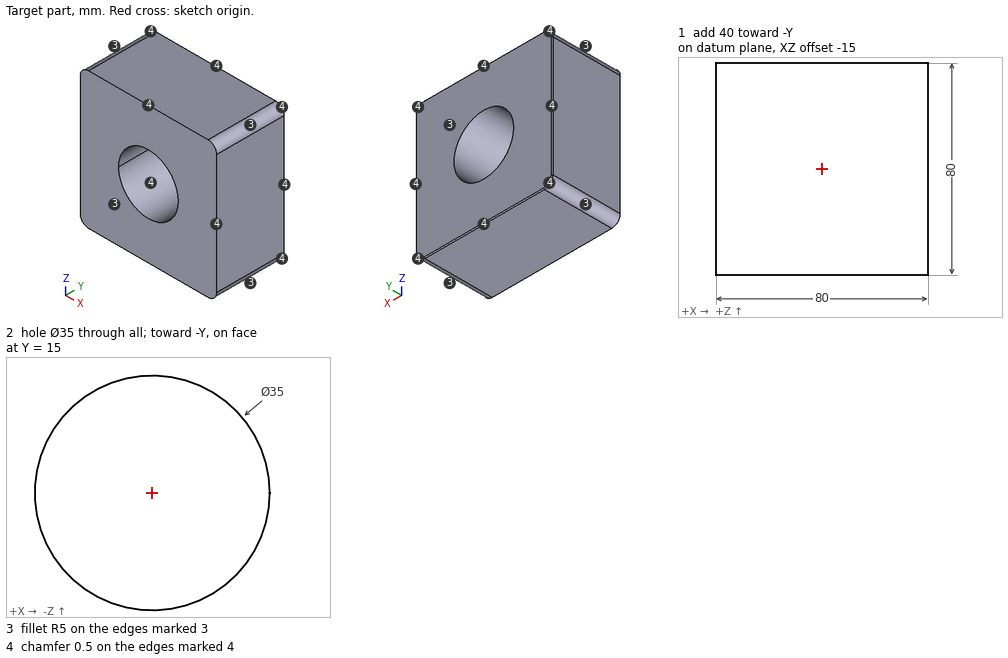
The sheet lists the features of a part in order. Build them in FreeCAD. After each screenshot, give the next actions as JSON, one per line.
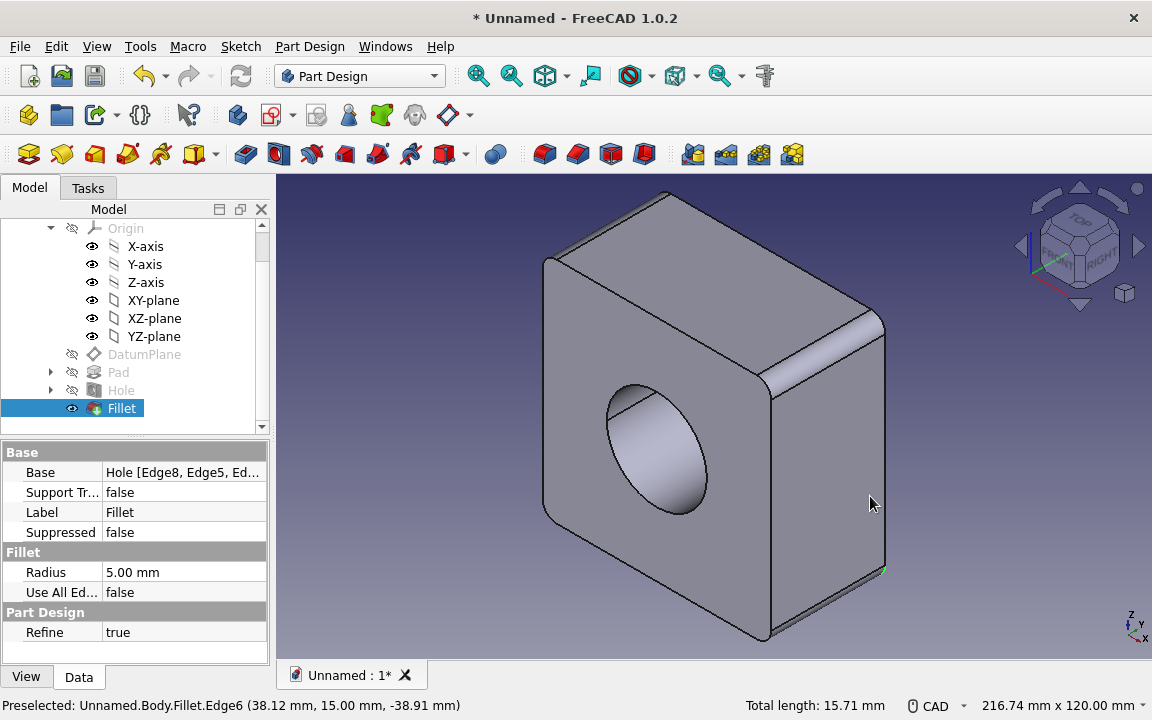
{"action": "left_click", "coordinate": [885, 327], "text": "ctrl"}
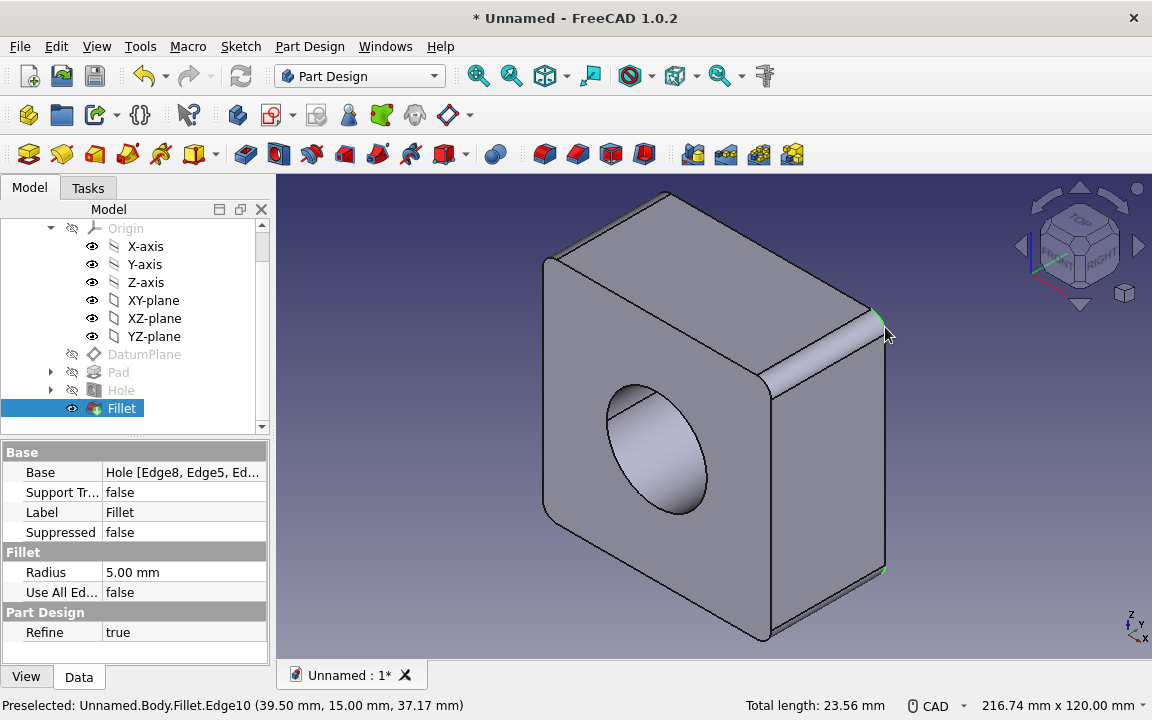
{"action": "key", "text": "2"}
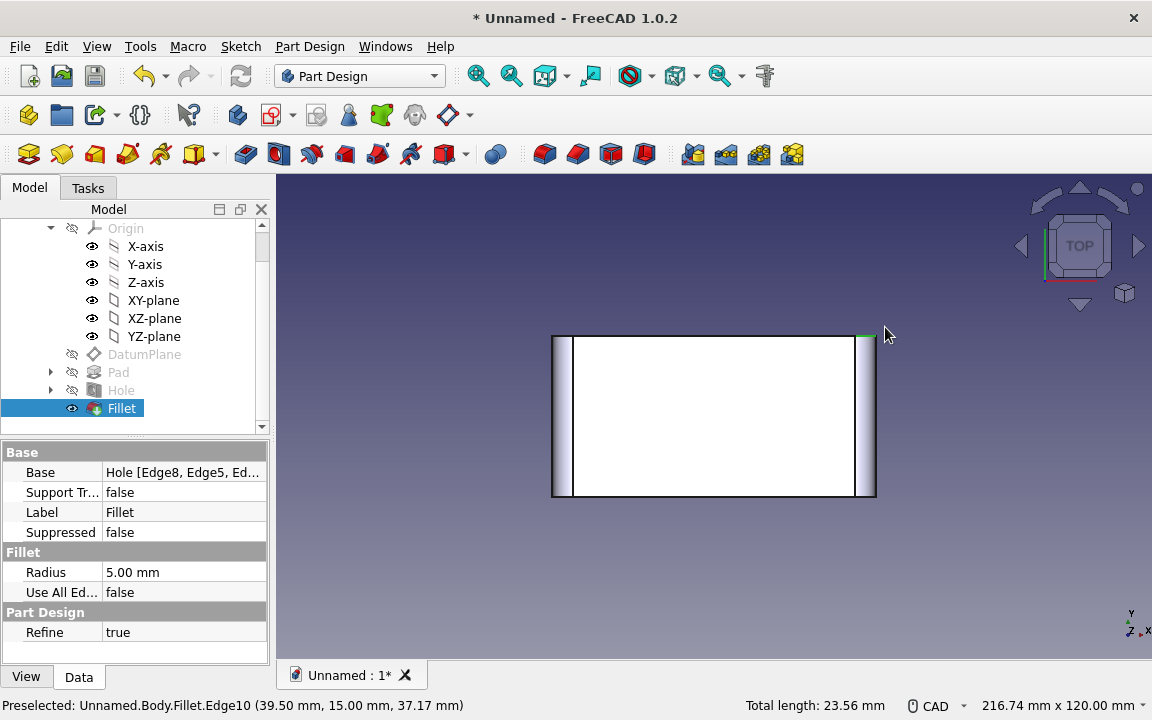
{"action": "left_click", "coordinate": [479, 76]}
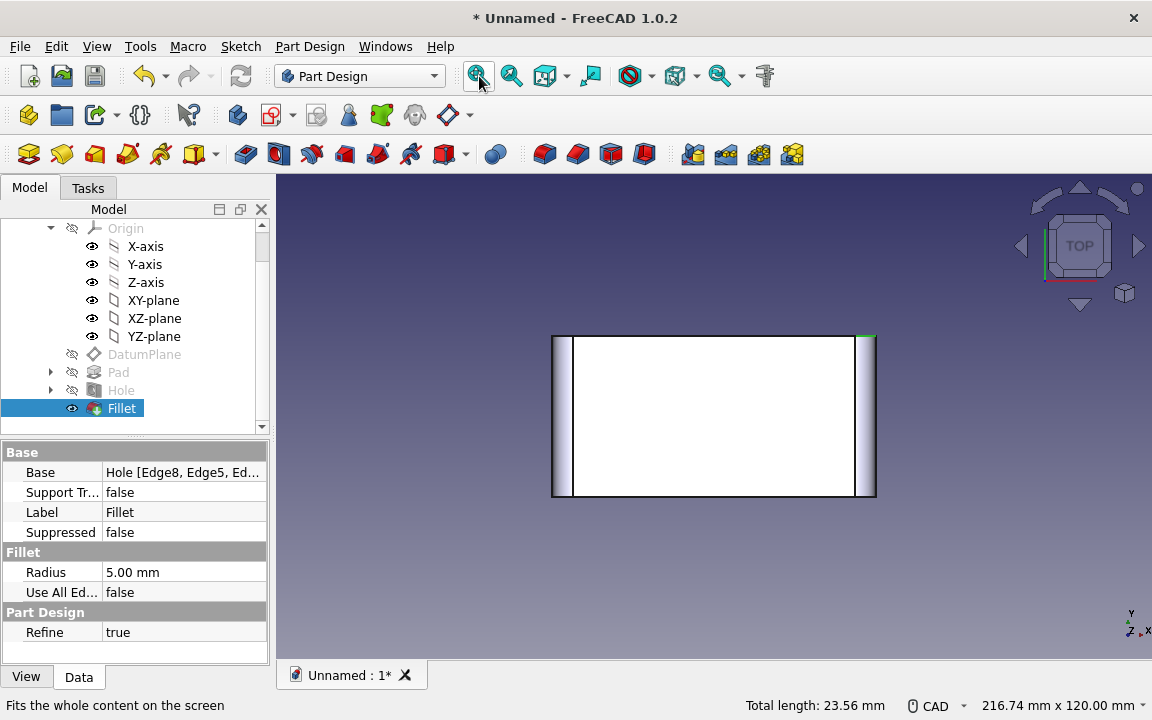
{"action": "left_click", "coordinate": [714, 335], "text": "ctrl"}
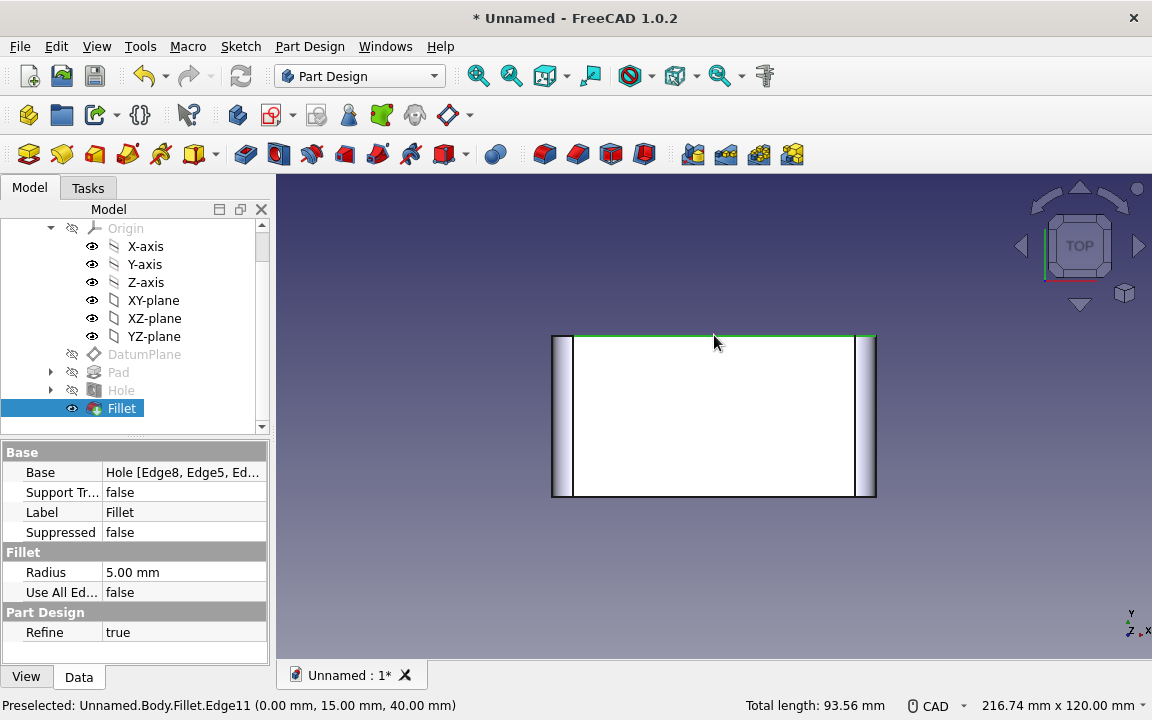
{"action": "left_click", "coordinate": [558, 335], "text": "ctrl"}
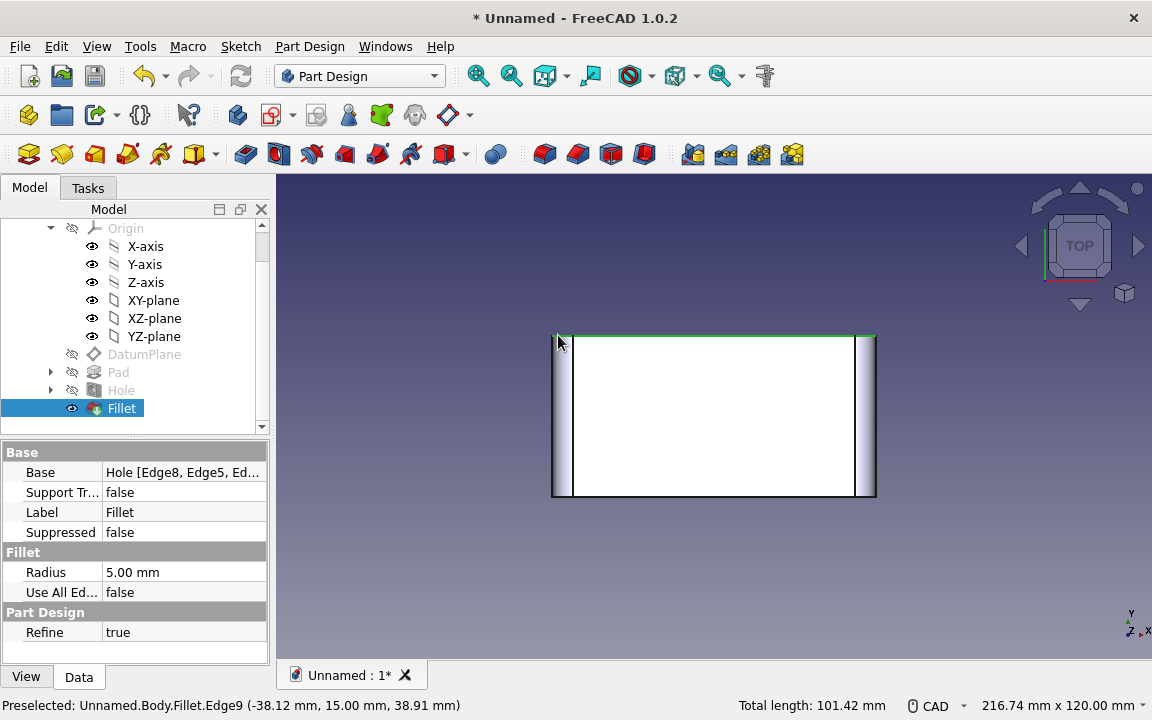
{"action": "key", "text": "1"}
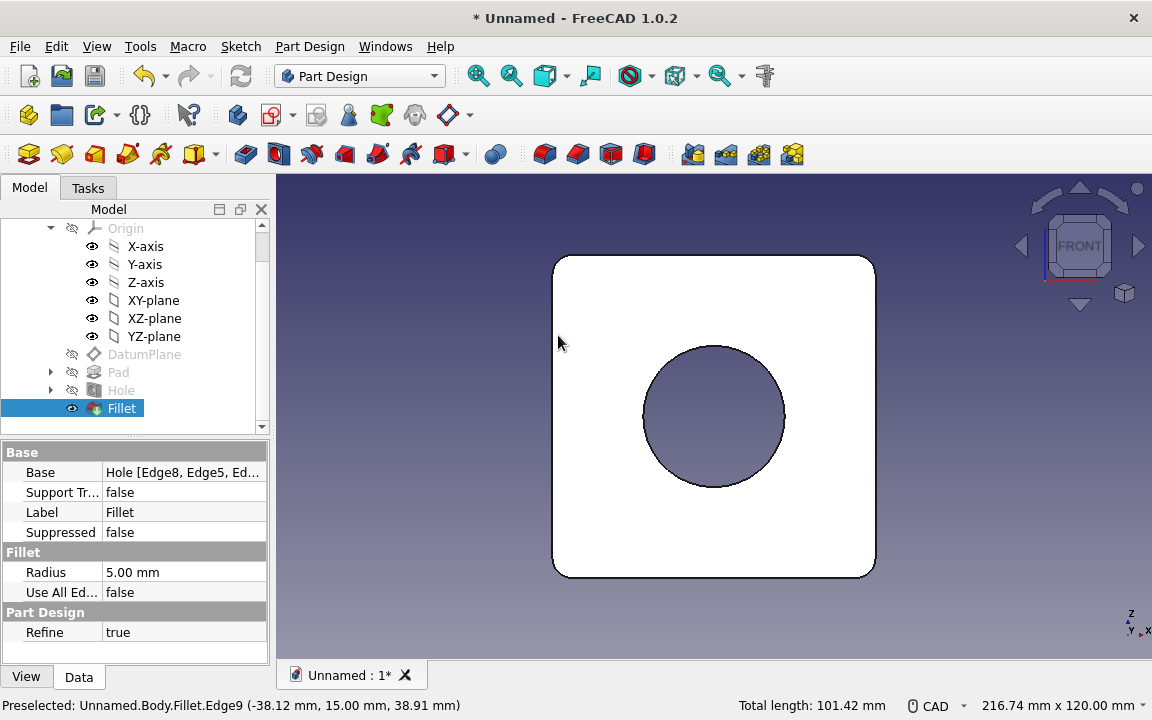
{"action": "key", "text": "3"}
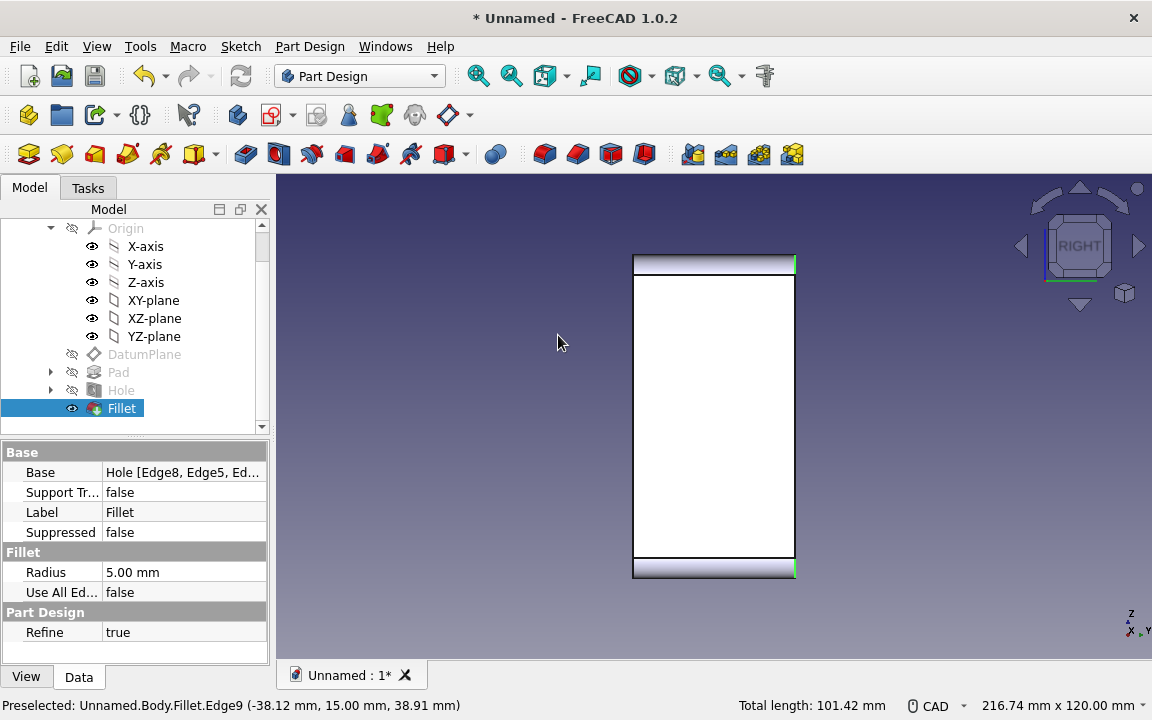
{"action": "left_click", "coordinate": [795, 415], "text": "ctrl"}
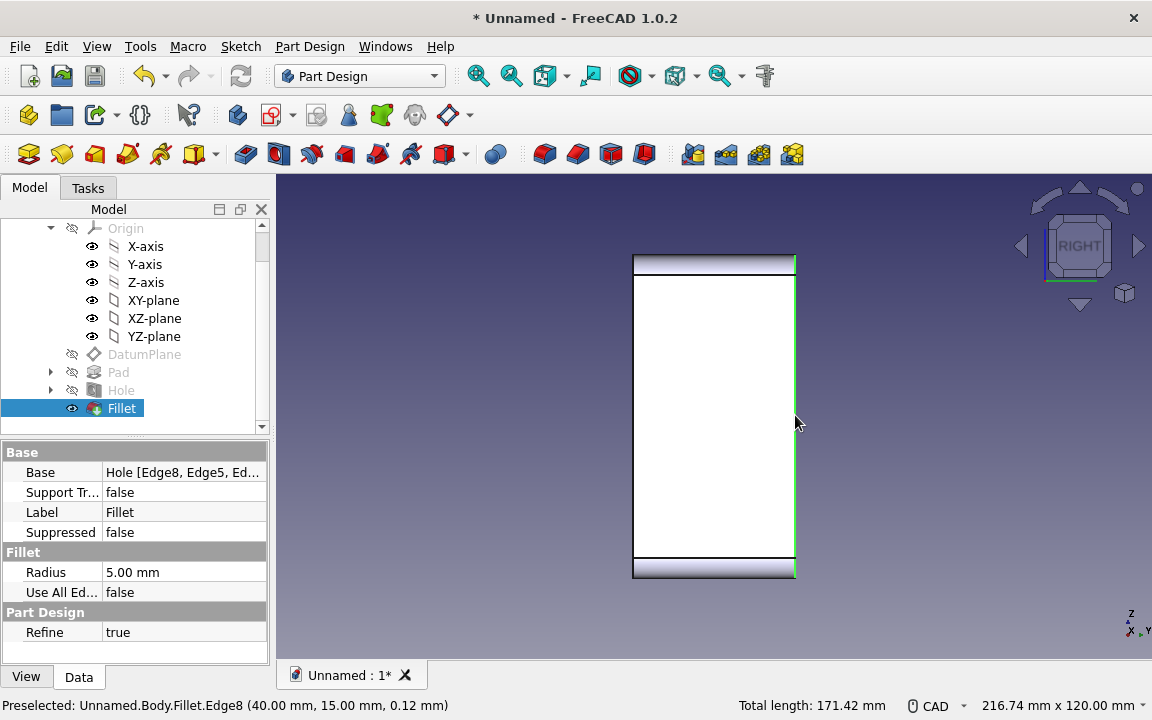
{"action": "key", "text": "5"}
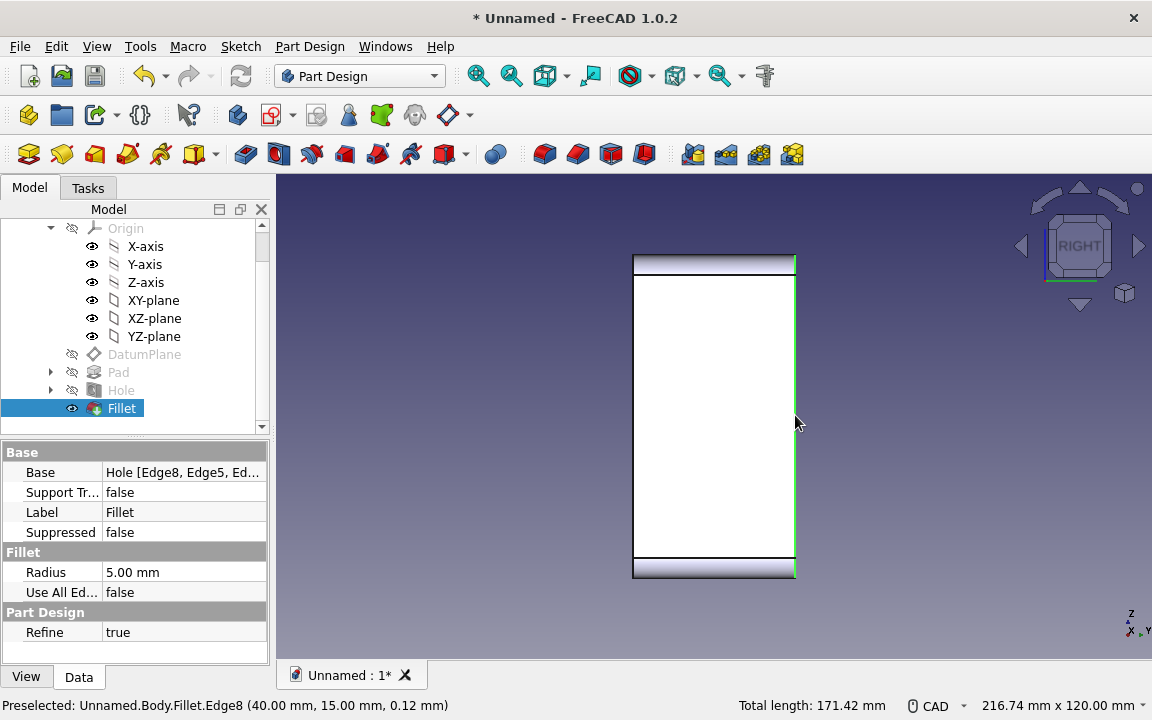
{"action": "left_click", "coordinate": [479, 76]}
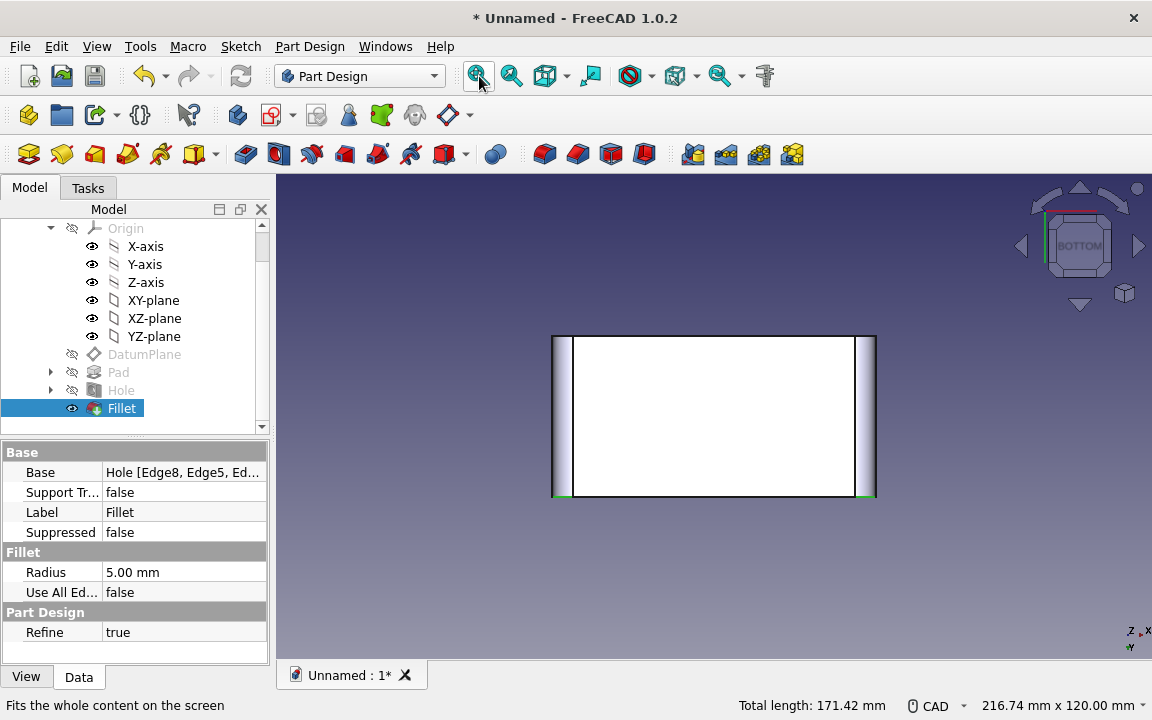
{"action": "key", "text": "4"}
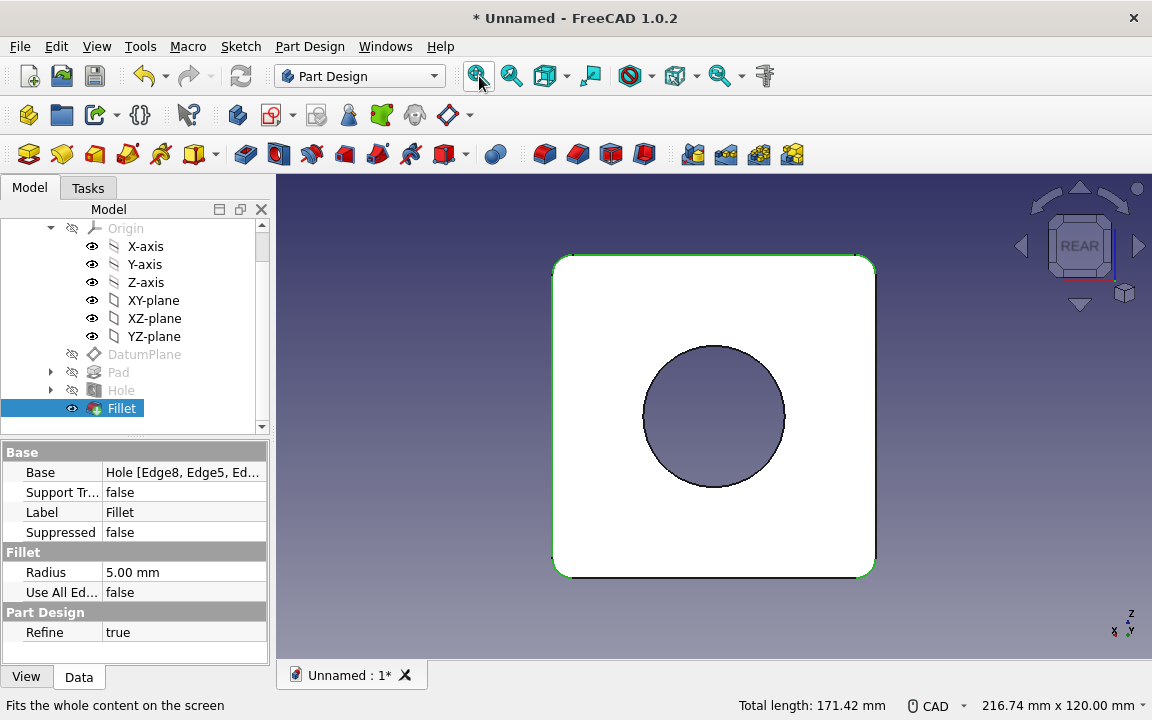
{"action": "left_click", "coordinate": [876, 416], "text": "ctrl"}